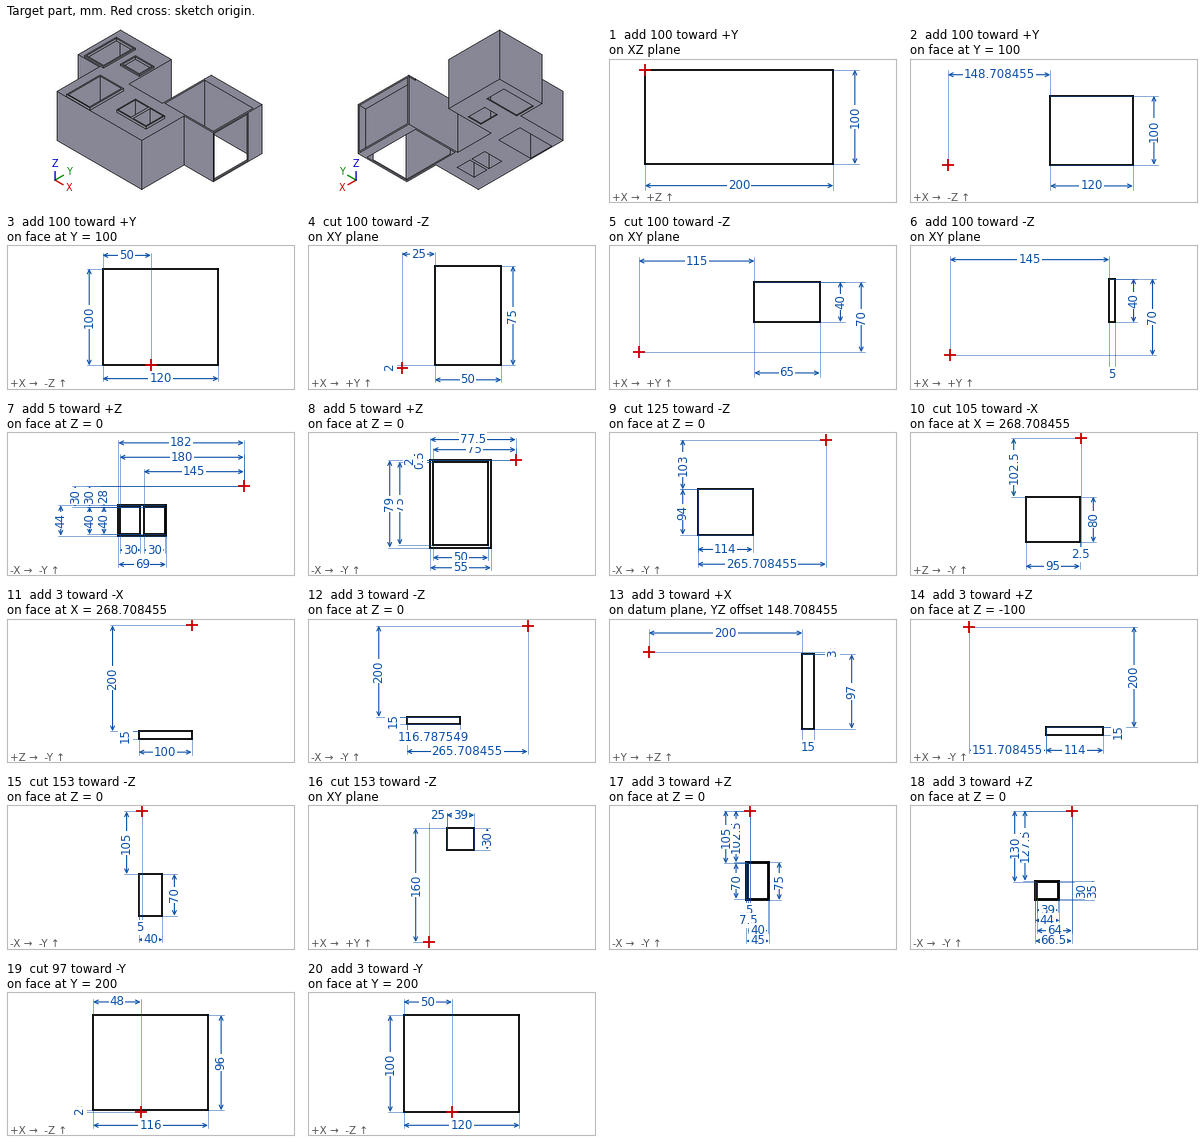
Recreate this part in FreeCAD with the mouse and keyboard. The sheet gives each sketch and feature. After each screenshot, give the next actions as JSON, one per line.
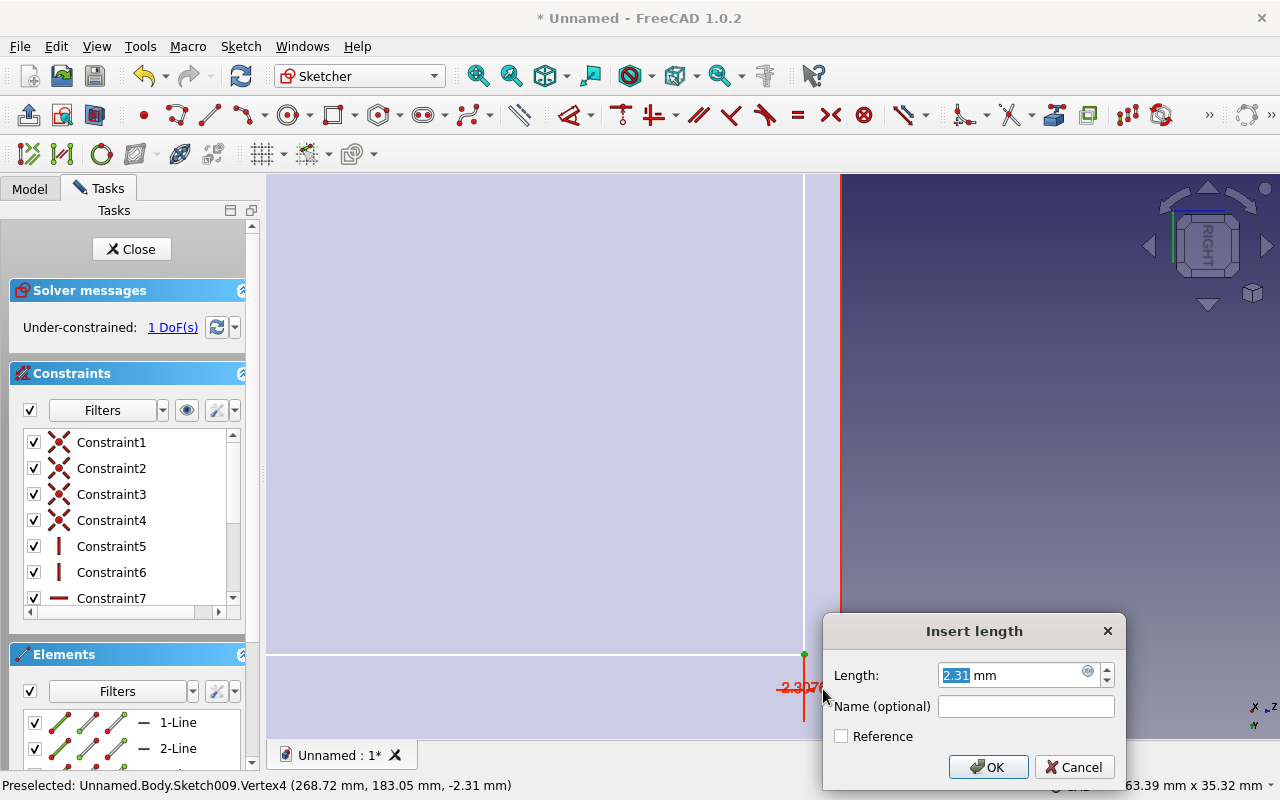
{"action": "type", "text": "2.5"}
{"action": "key", "text": "Return"}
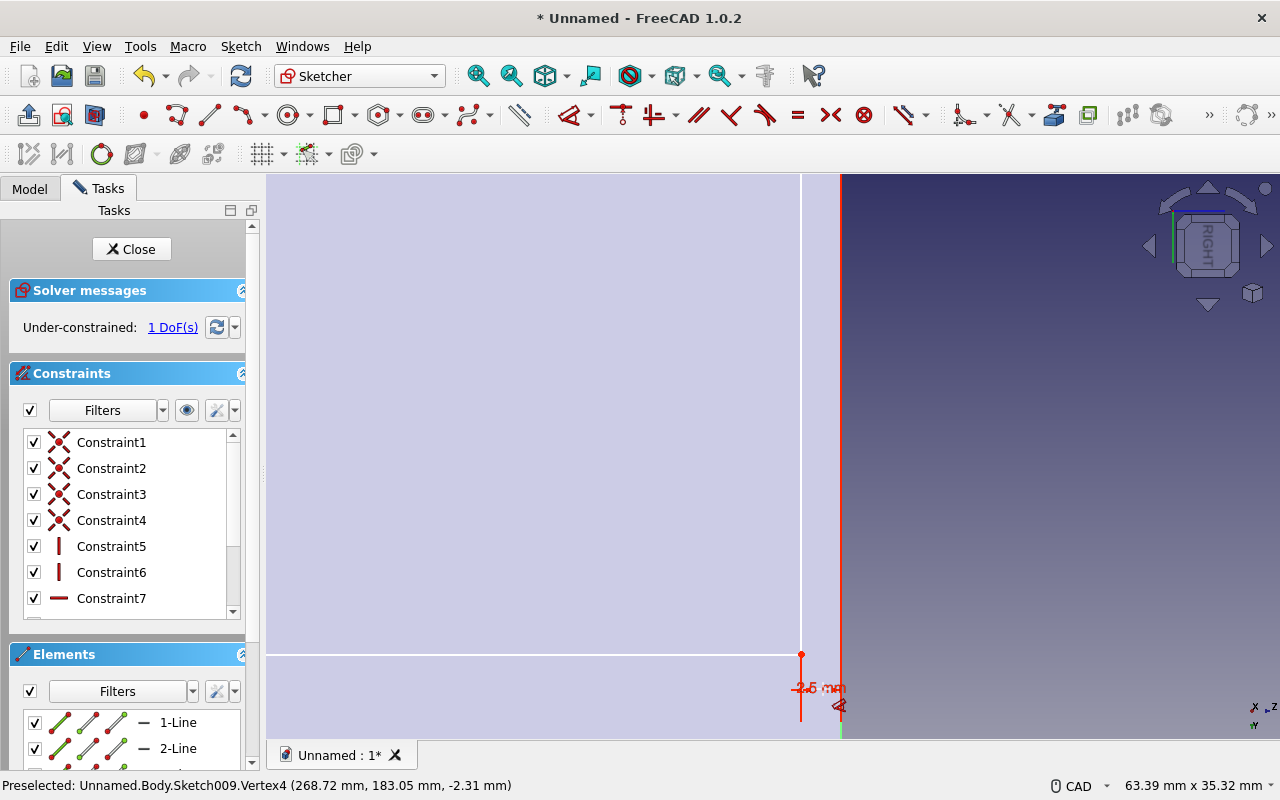
{"action": "scroll", "coordinate": [805, 655], "scroll_direction": "down", "scroll_amount": 10}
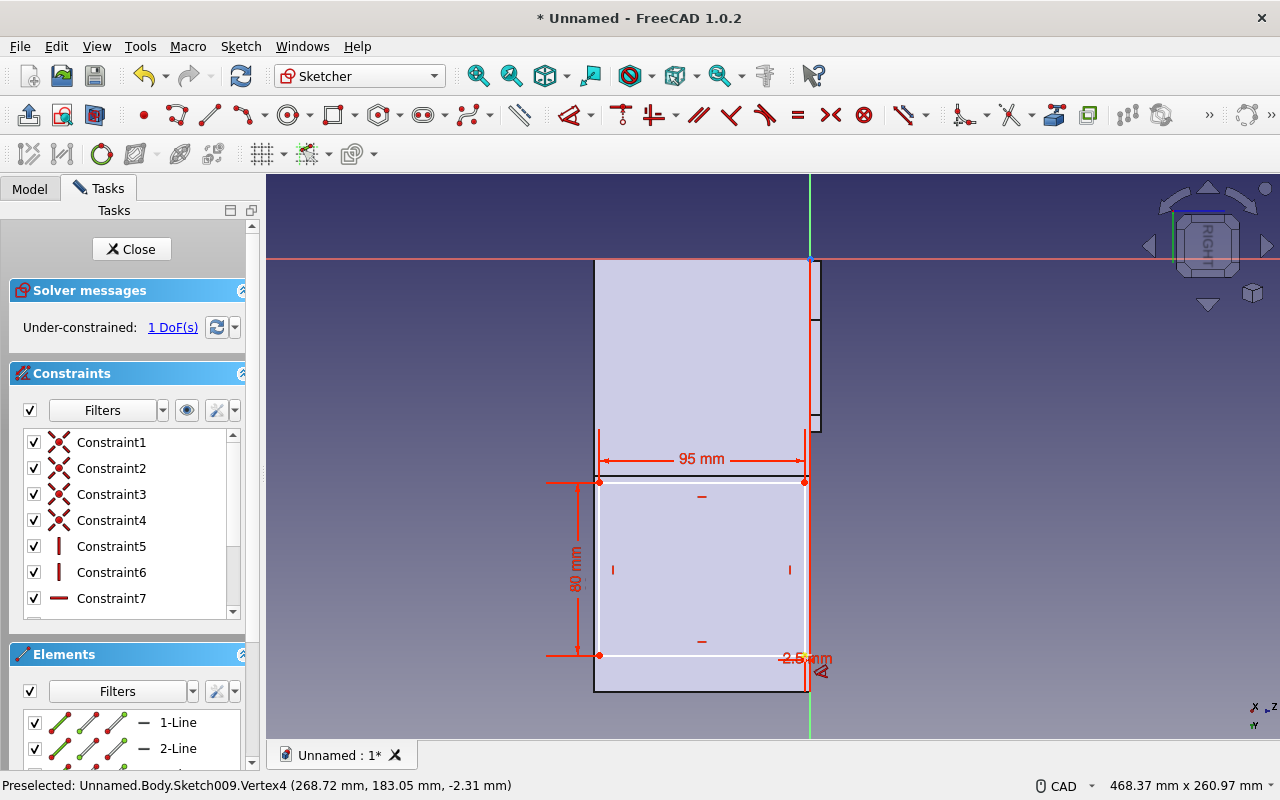
{"action": "left_click", "coordinate": [599, 483]}
{"action": "left_click", "coordinate": [565, 371]}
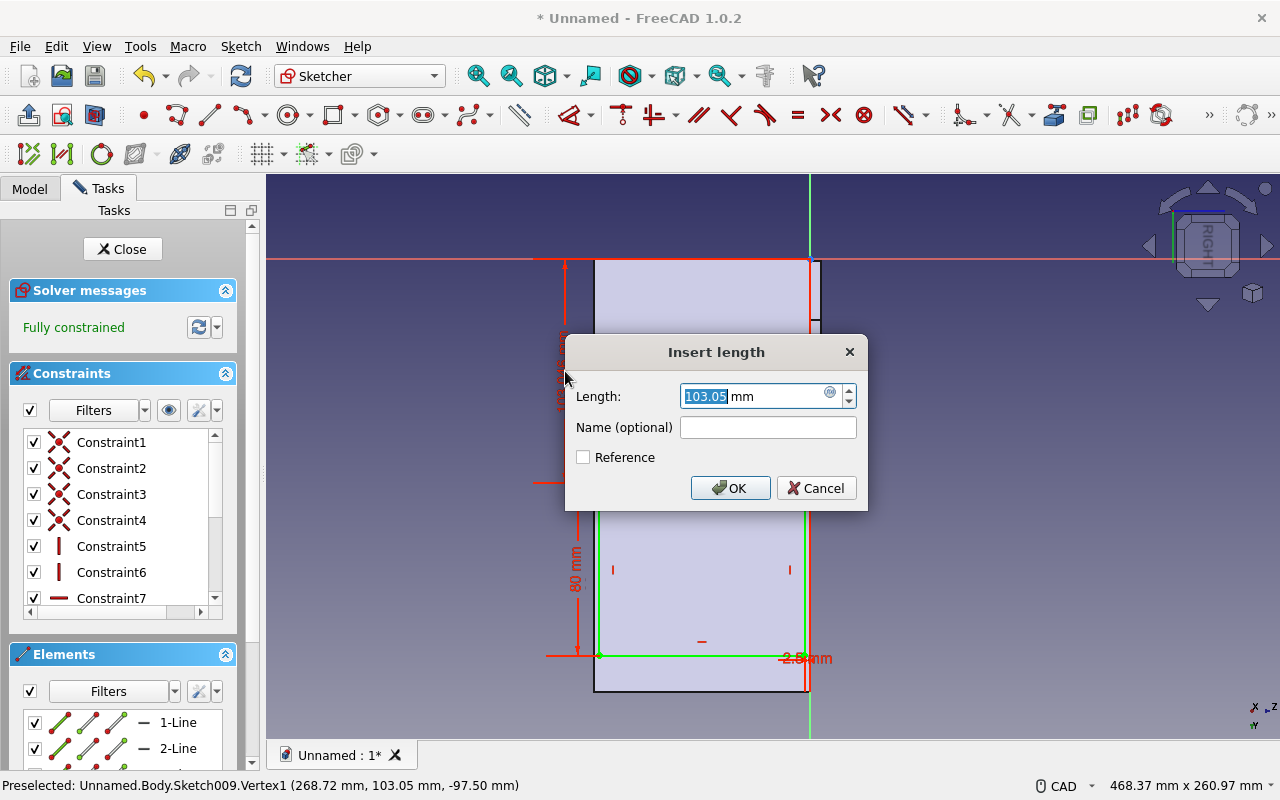
{"action": "type", "text": "102.5"}
{"action": "key", "text": "Return"}
{"action": "key", "text": "Escape"}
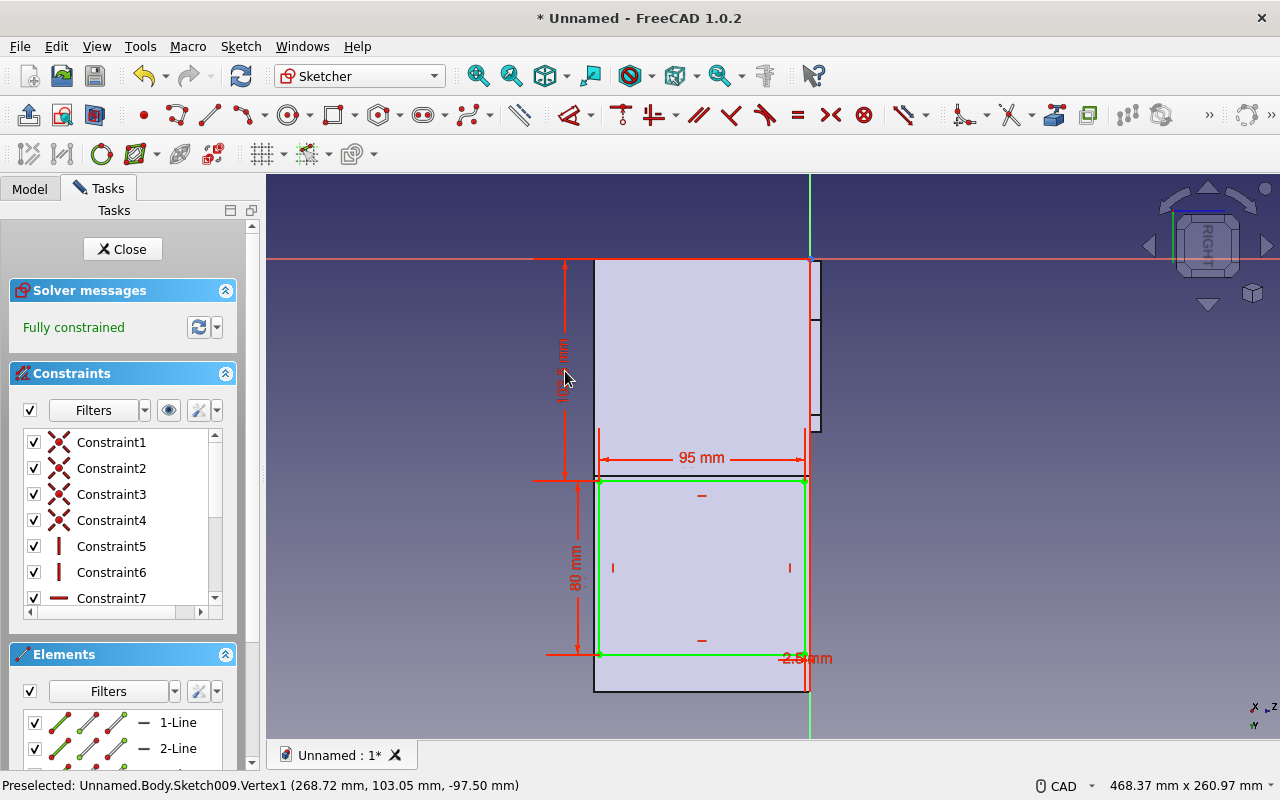
{"action": "left_click", "coordinate": [123, 249]}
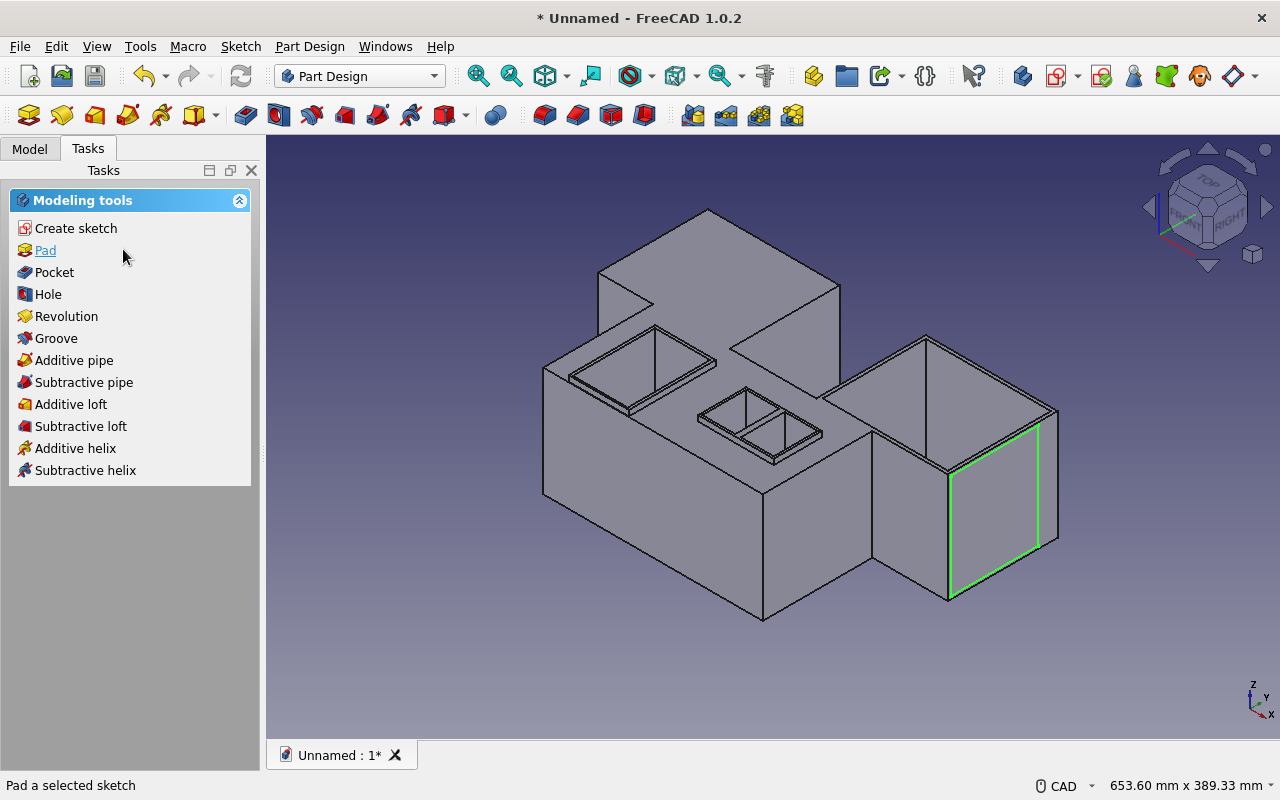
{"action": "left_click", "coordinate": [246, 116]}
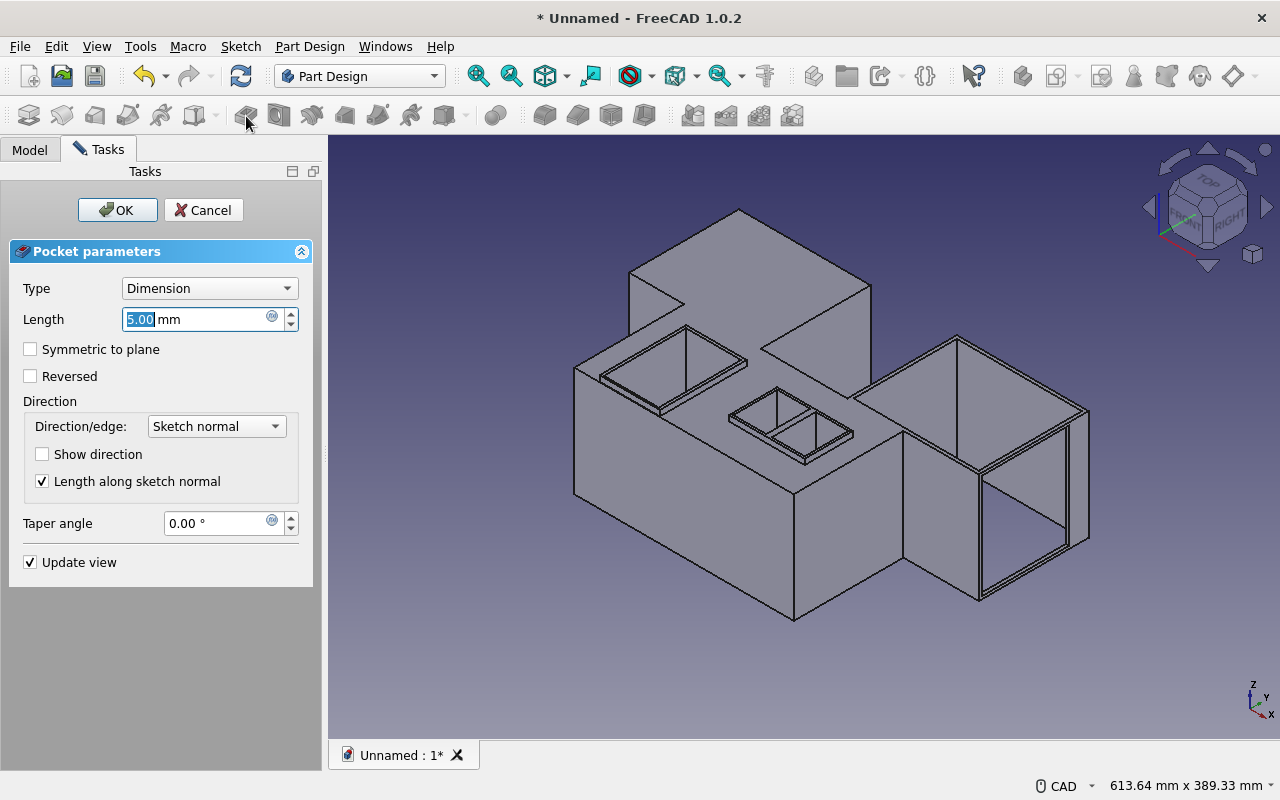
{"action": "type", "text": "105"}
{"action": "key", "text": "Tab"}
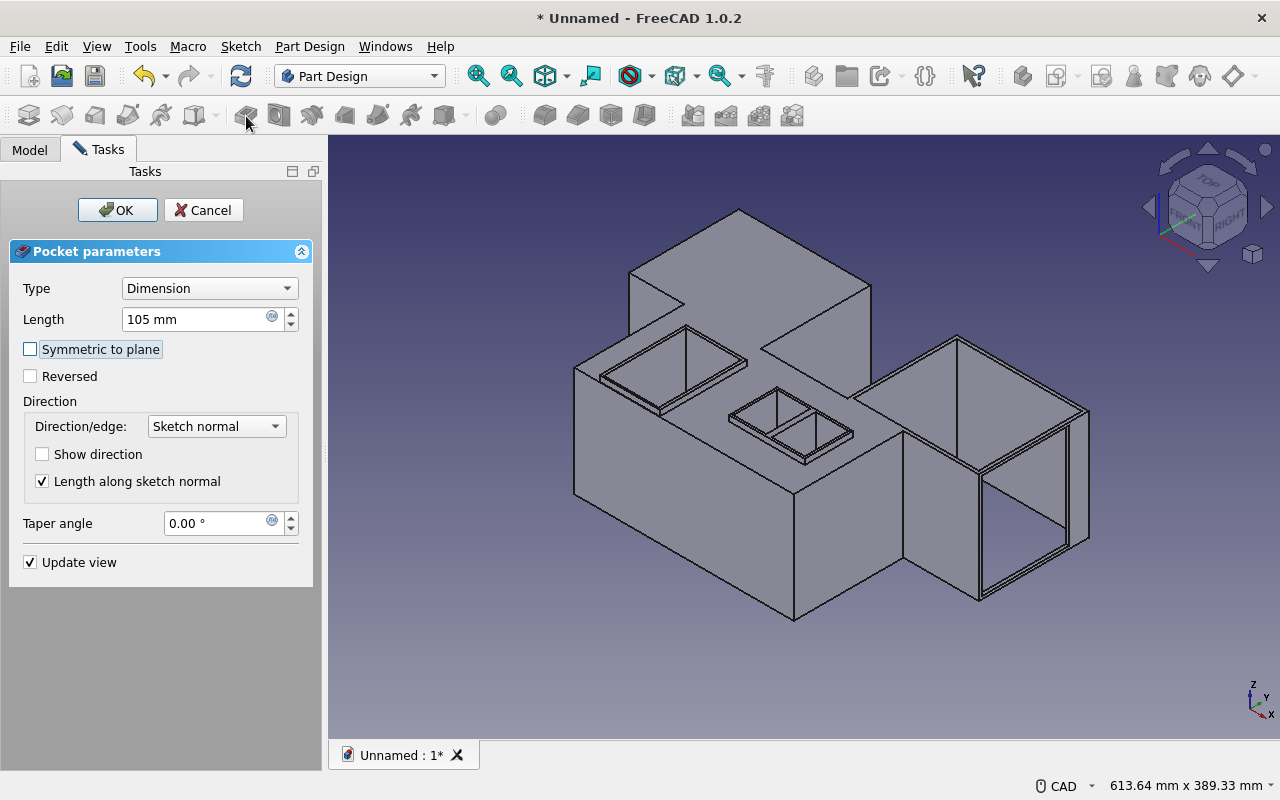
{"action": "left_click", "coordinate": [118, 210]}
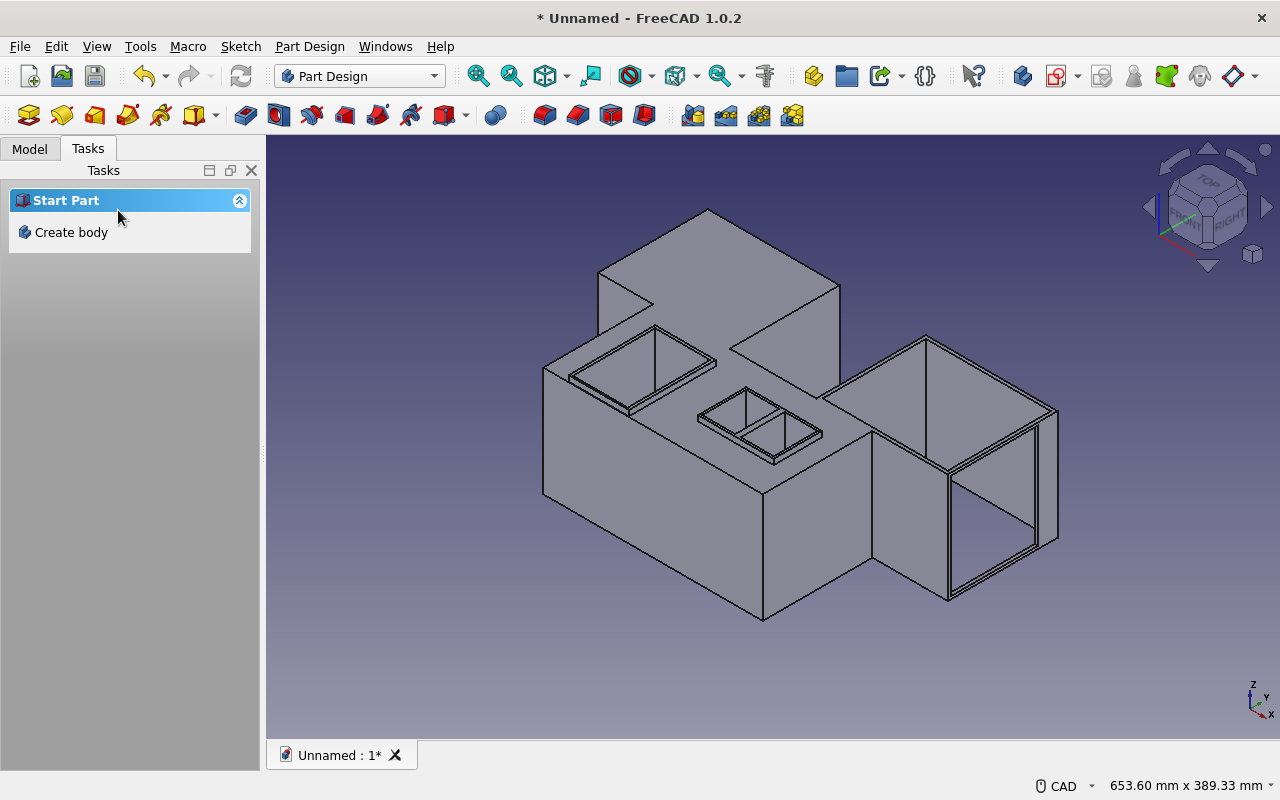
{"action": "left_click", "coordinate": [1050, 496]}